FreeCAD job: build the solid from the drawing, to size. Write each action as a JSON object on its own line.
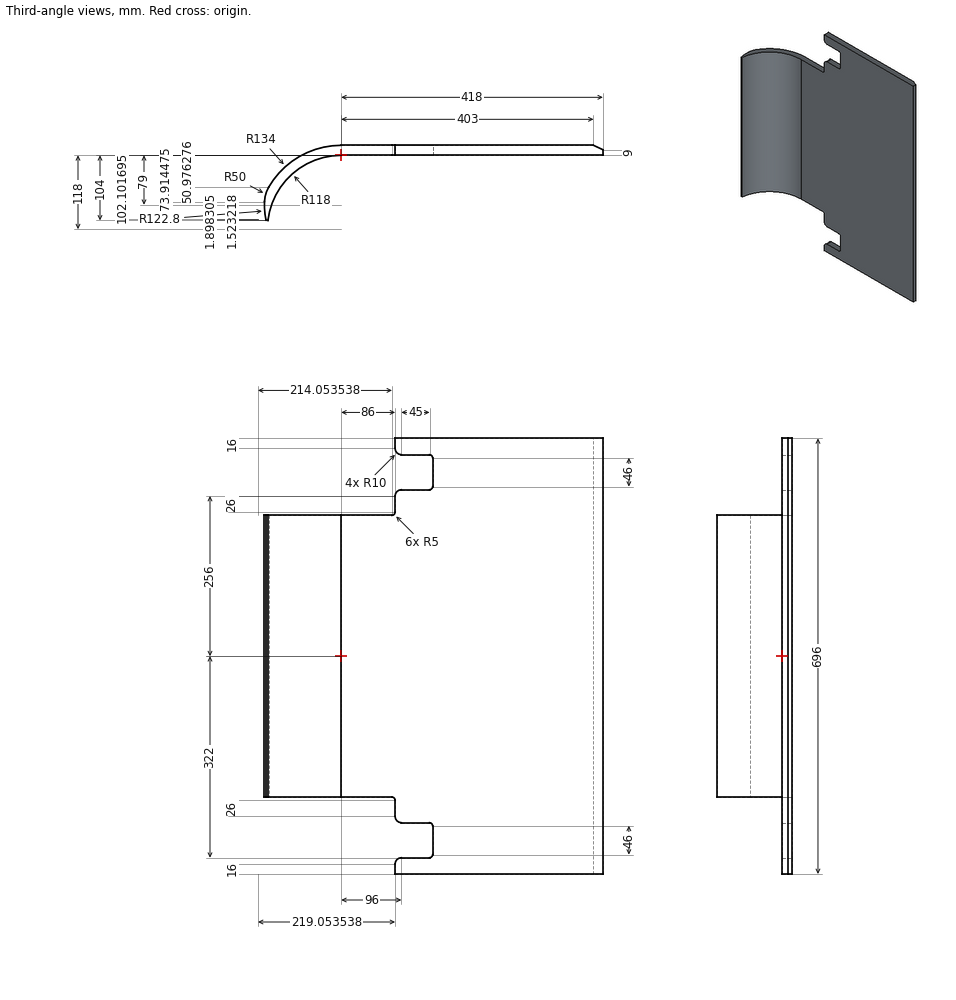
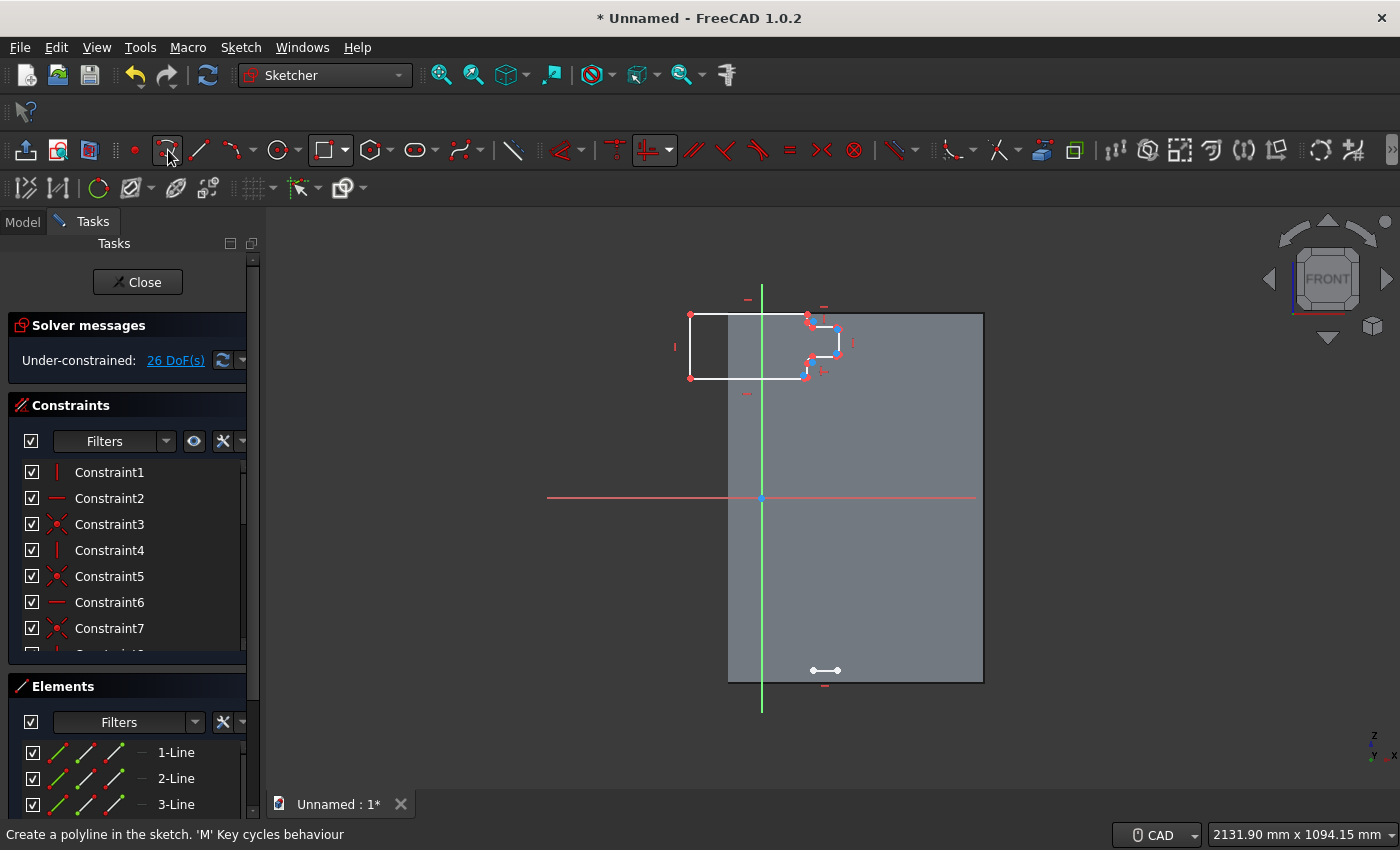
{"action": "scroll", "coordinate": [807, 675], "scroll_direction": "up", "scroll_amount": 4}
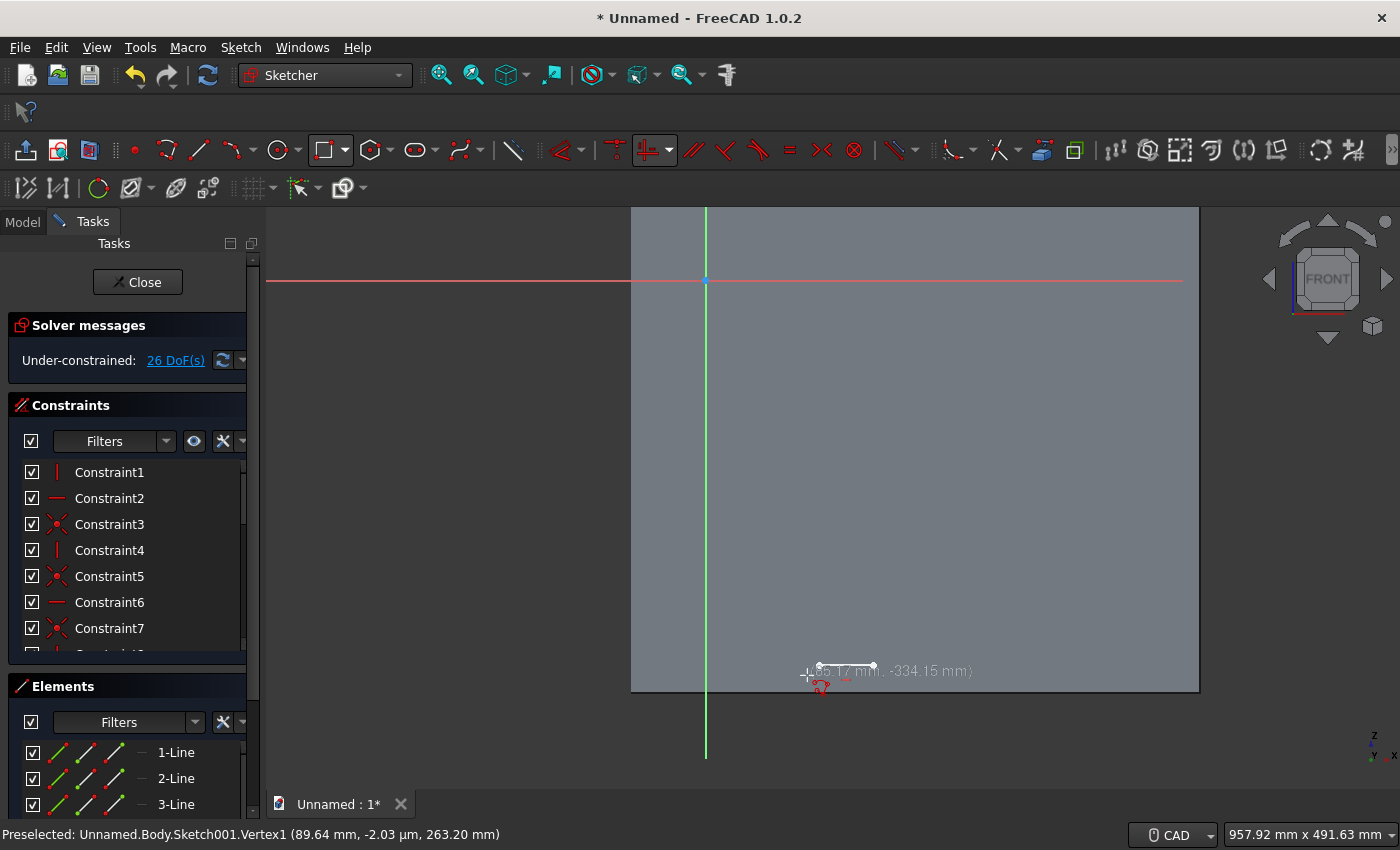
{"action": "left_click", "coordinate": [807, 674]}
{"action": "left_click", "coordinate": [807, 693]}
{"action": "left_click", "coordinate": [548, 693]}
{"action": "left_click", "coordinate": [548, 547]}
{"action": "left_click", "coordinate": [801, 547]}
{"action": "right_click", "coordinate": [801, 547]}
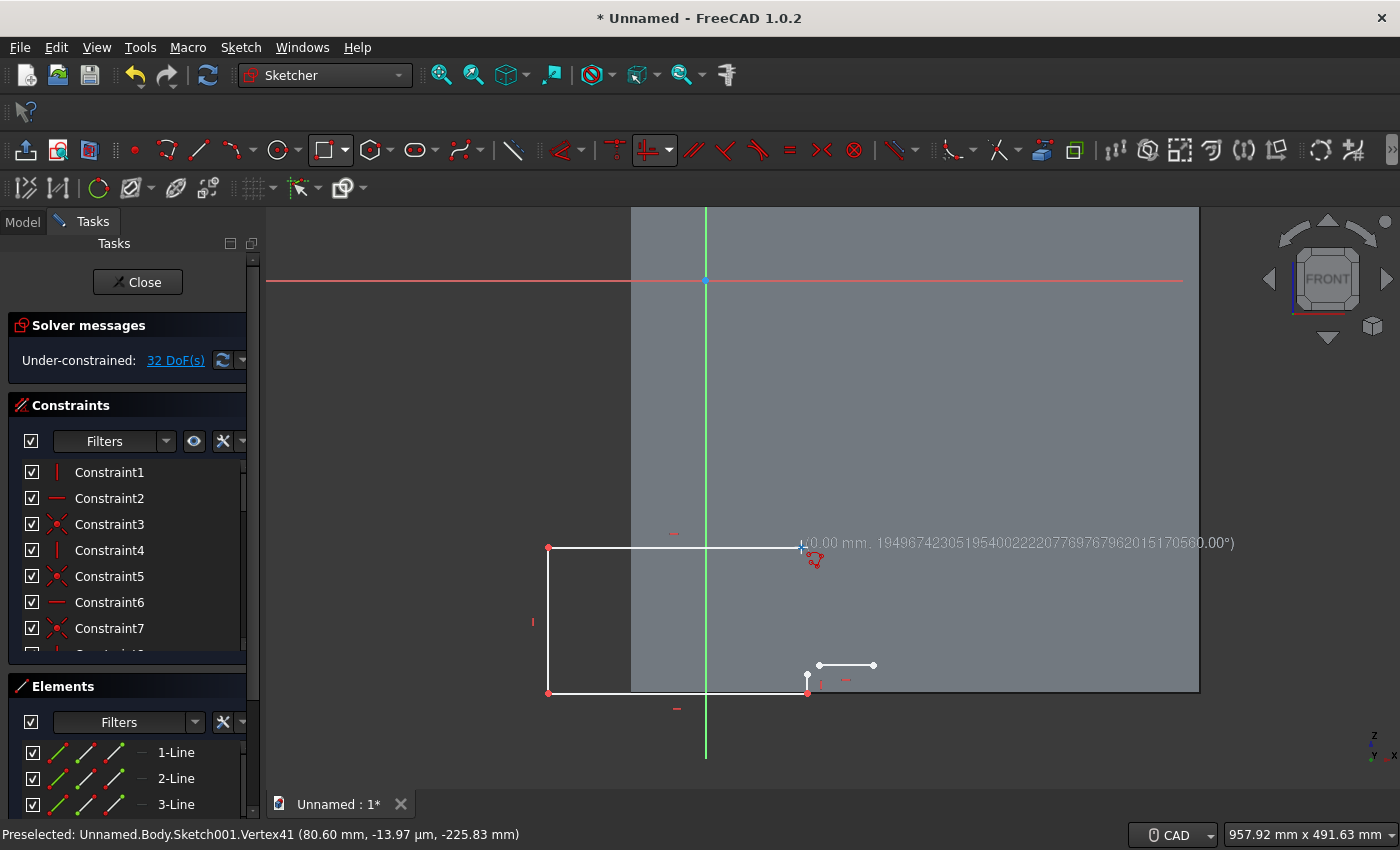
{"action": "left_click", "coordinate": [200, 150]}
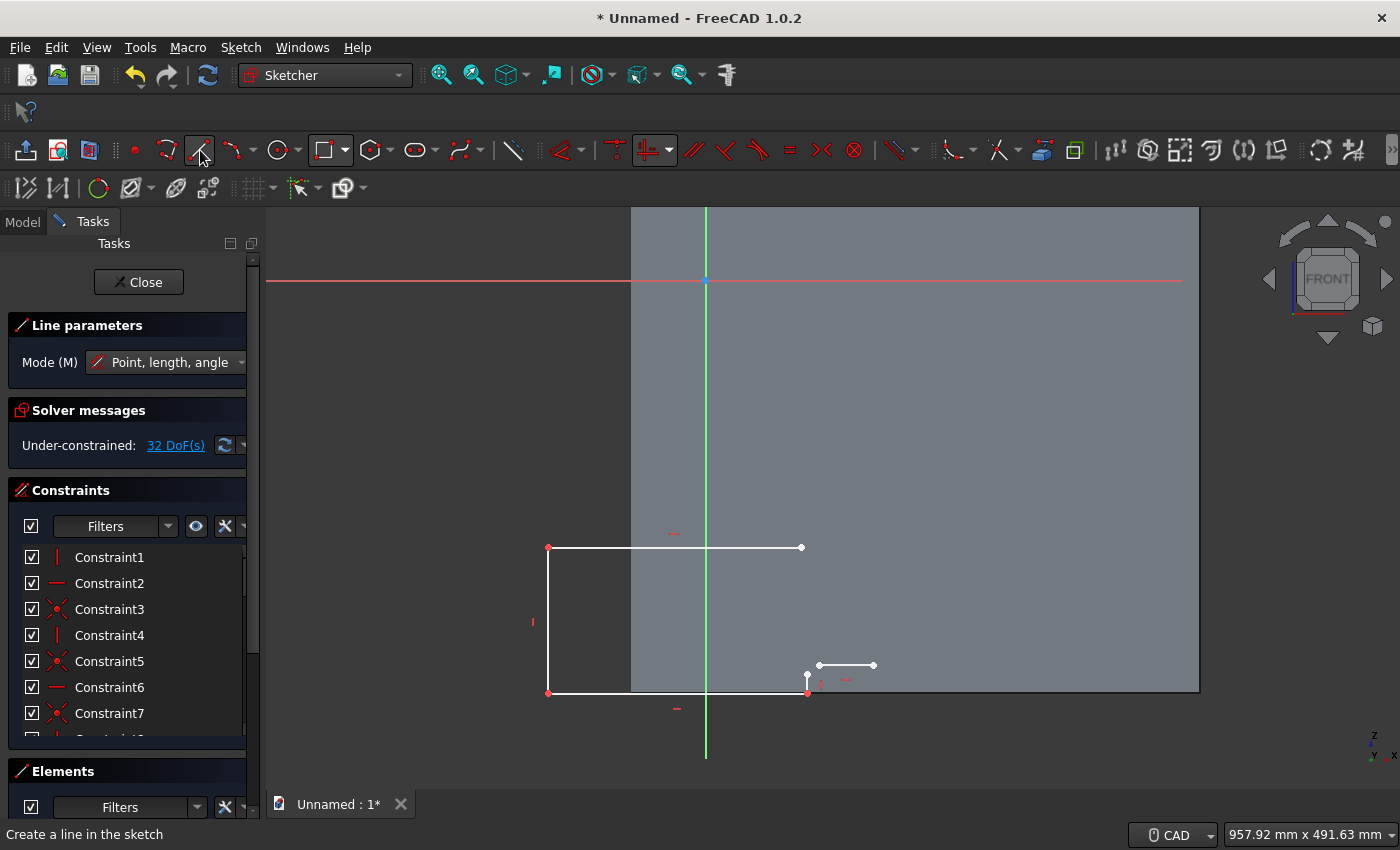
{"action": "scroll", "coordinate": [807, 553], "scroll_direction": "up", "scroll_amount": 4}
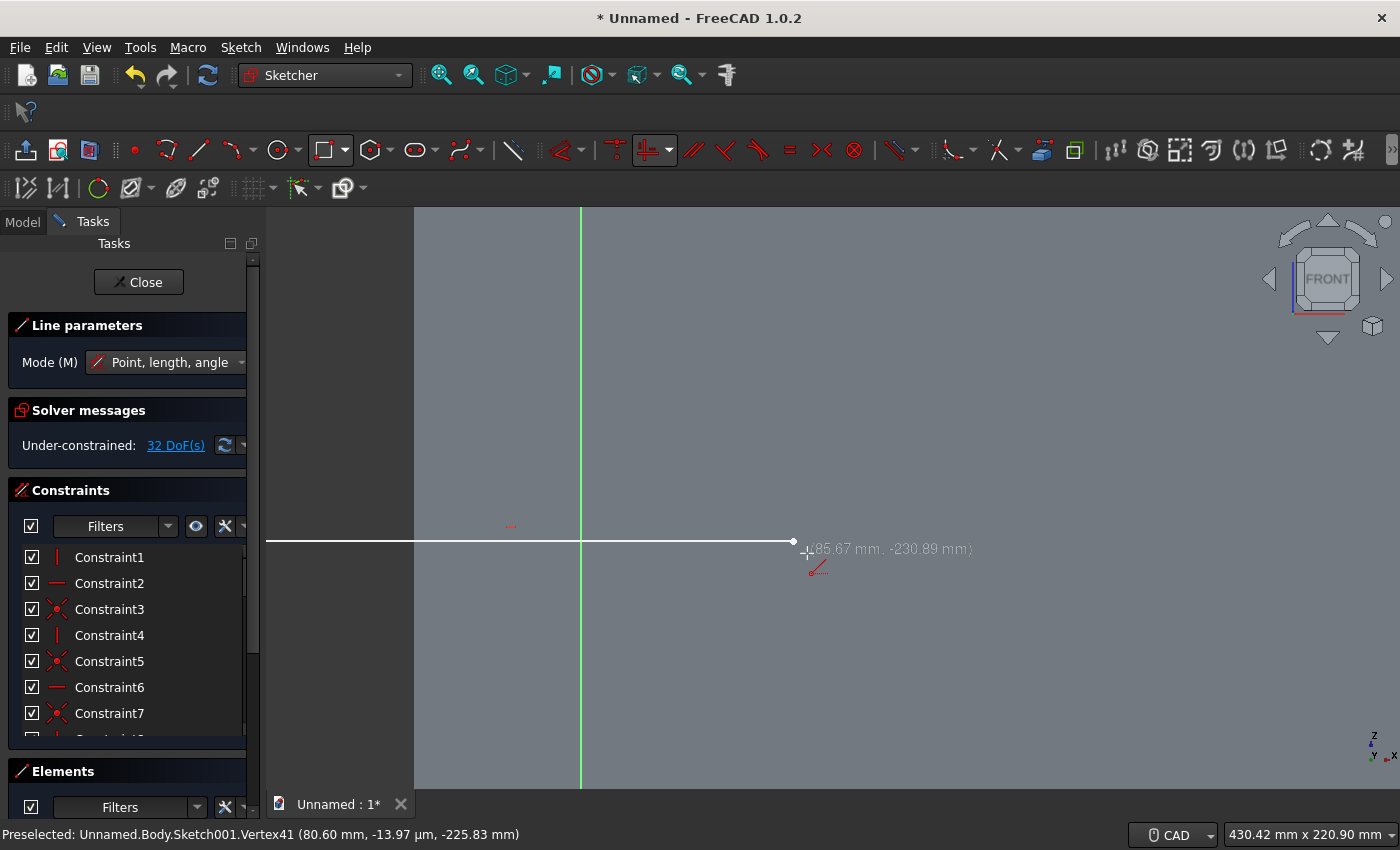
{"action": "left_click", "coordinate": [807, 552]}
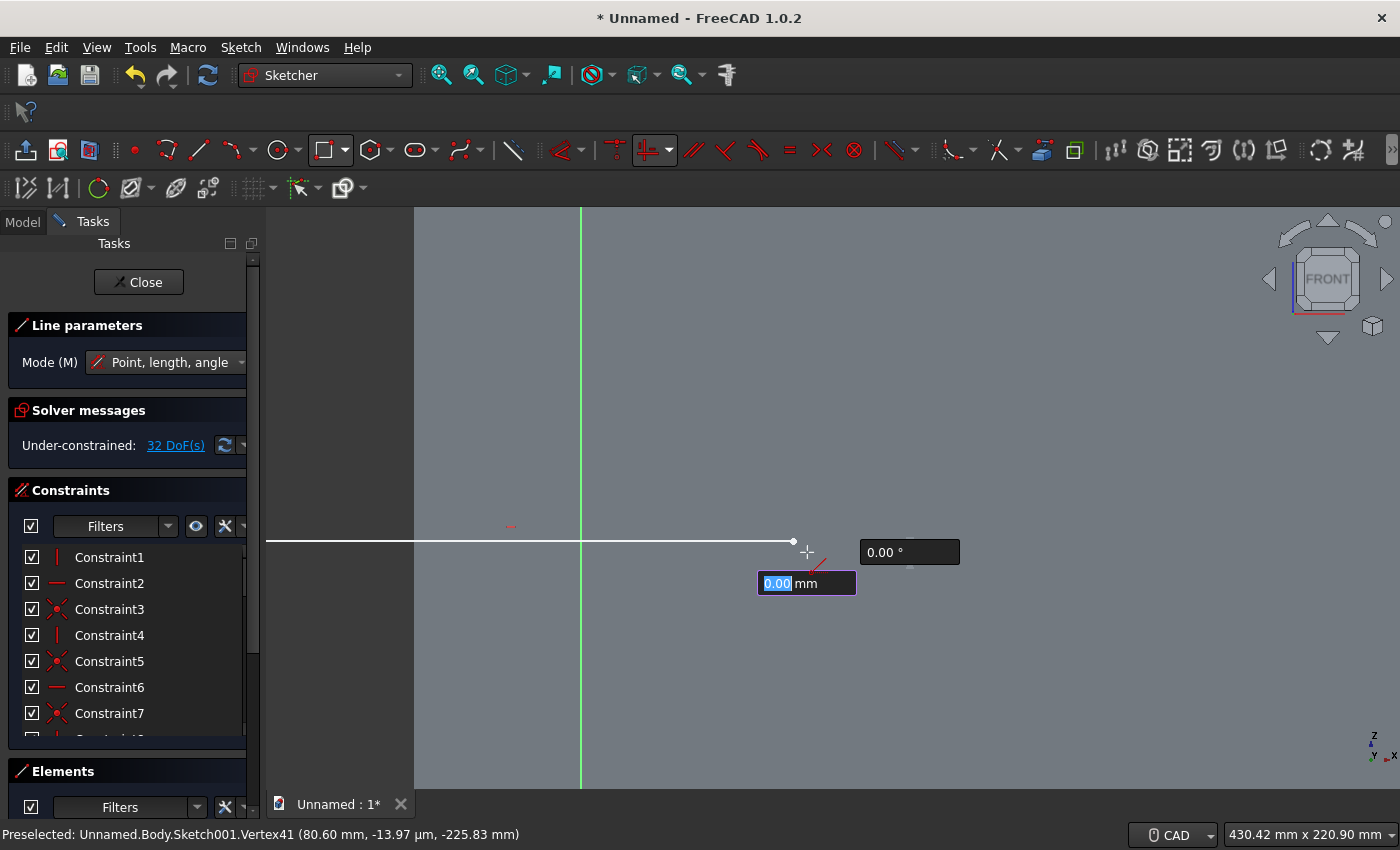
{"action": "scroll", "coordinate": [807, 638], "scroll_direction": "down", "scroll_amount": 8}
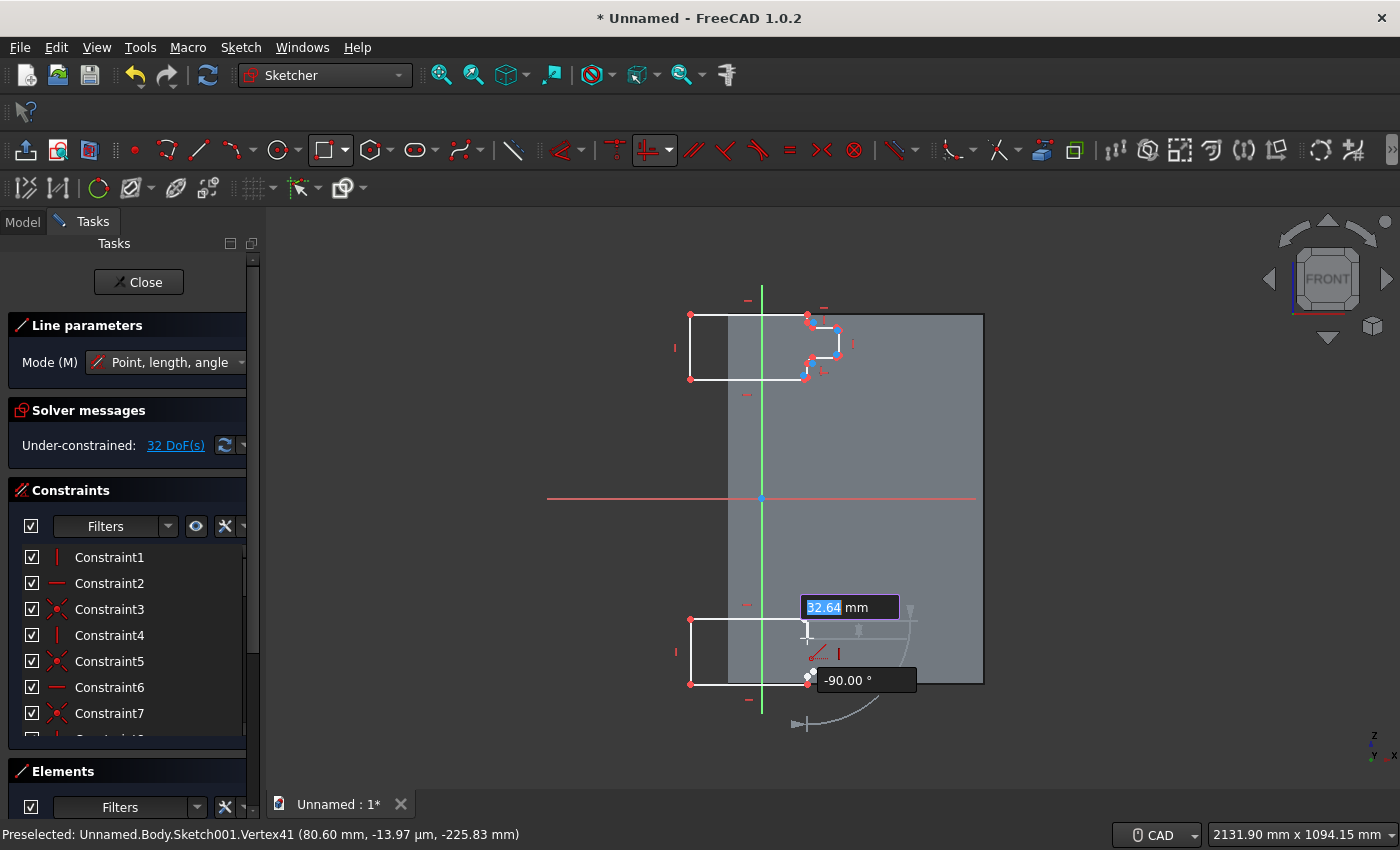
{"action": "left_click", "coordinate": [807, 635]}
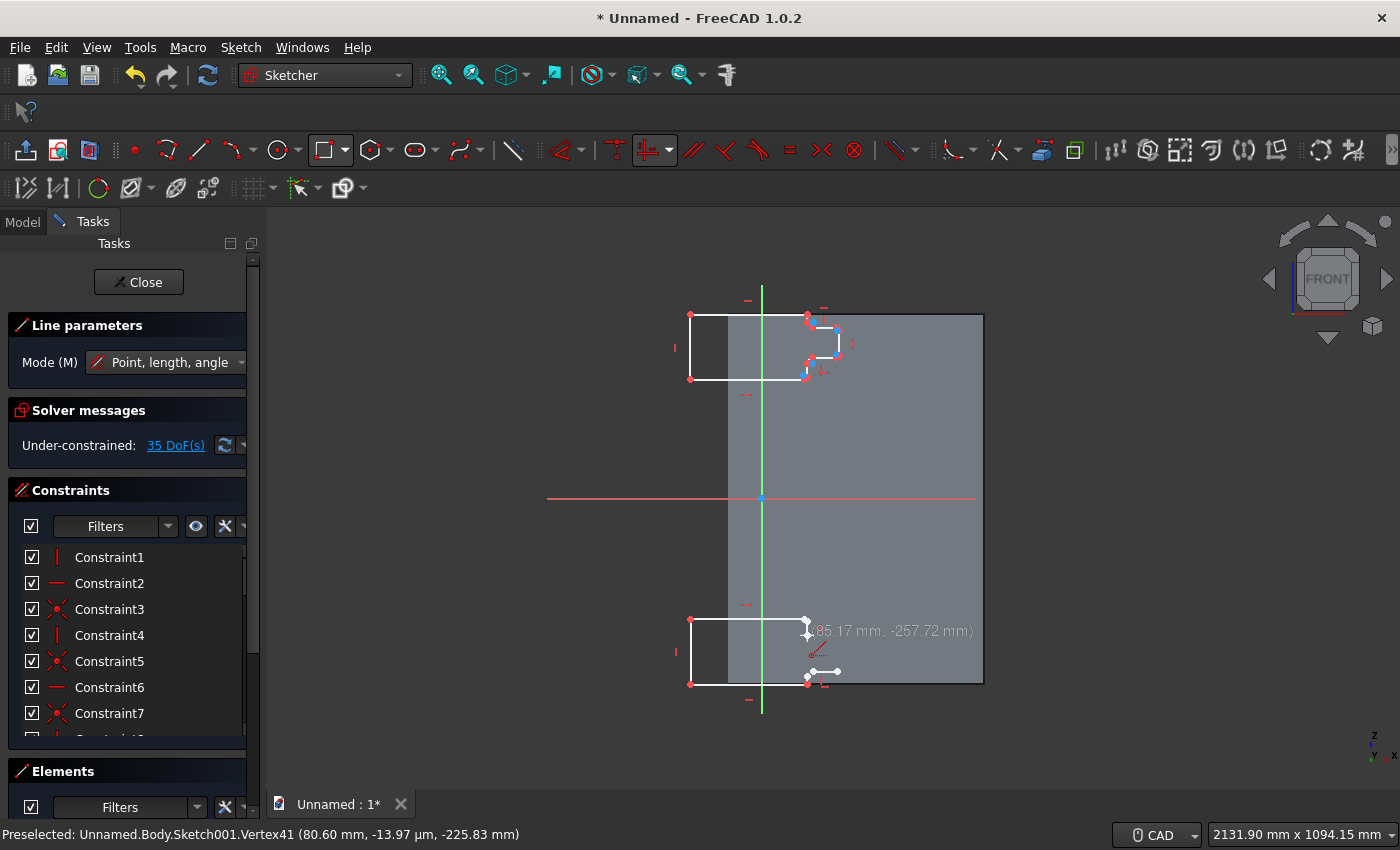
{"action": "scroll", "coordinate": [813, 640], "scroll_direction": "up", "scroll_amount": 4}